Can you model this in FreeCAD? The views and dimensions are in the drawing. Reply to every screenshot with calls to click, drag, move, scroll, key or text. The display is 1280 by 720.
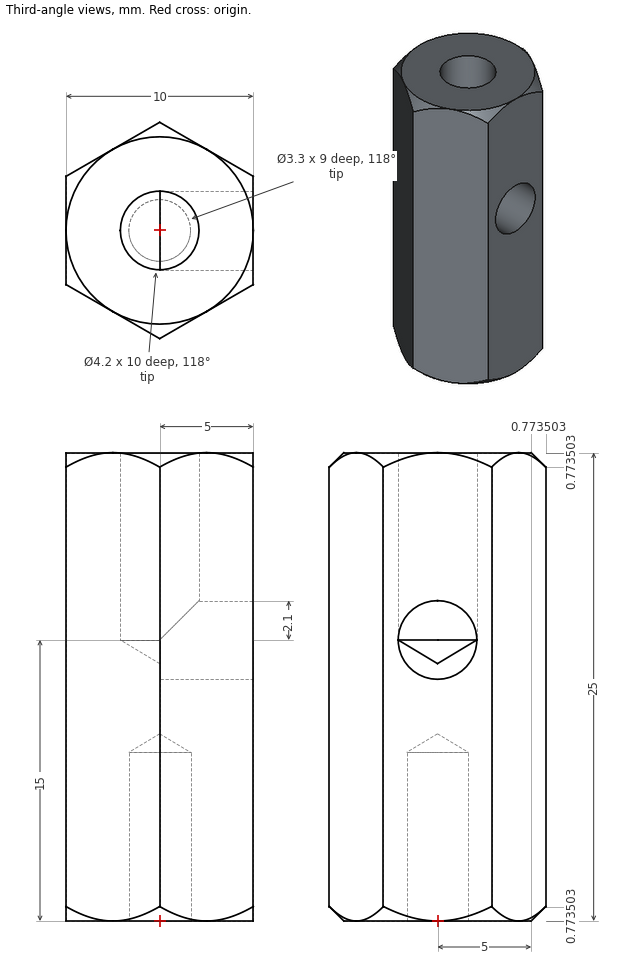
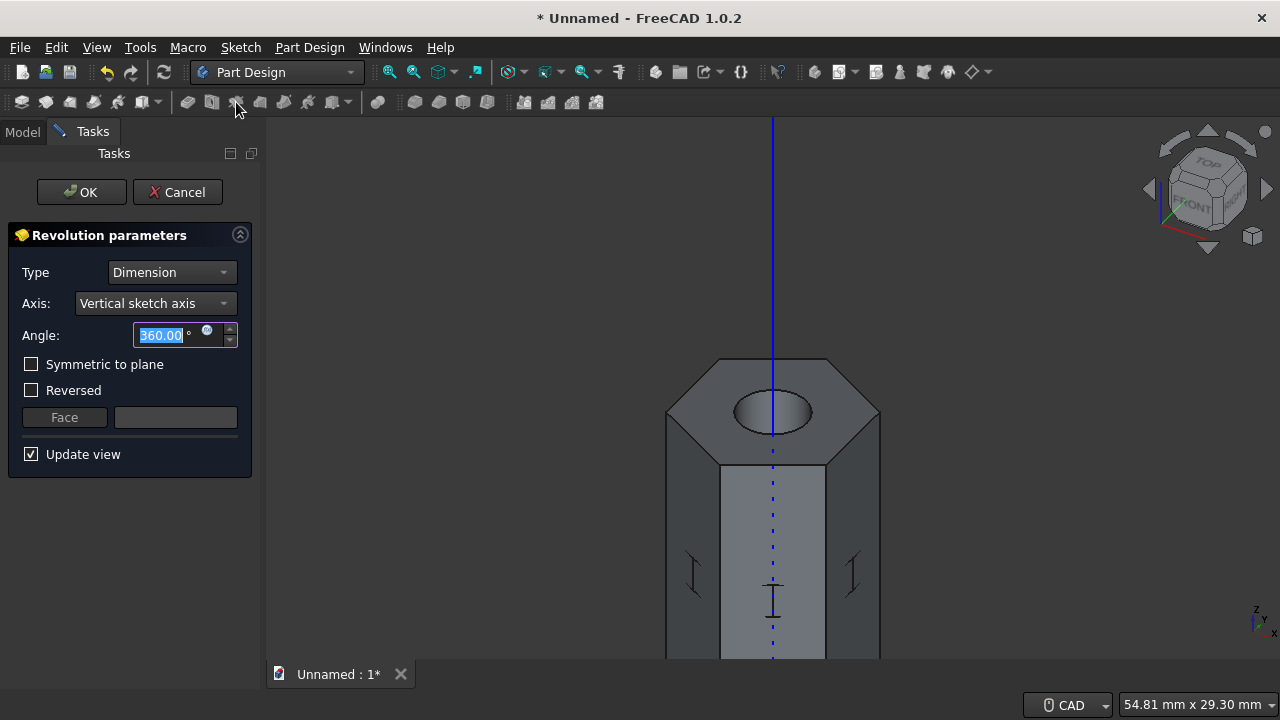
click(156, 304)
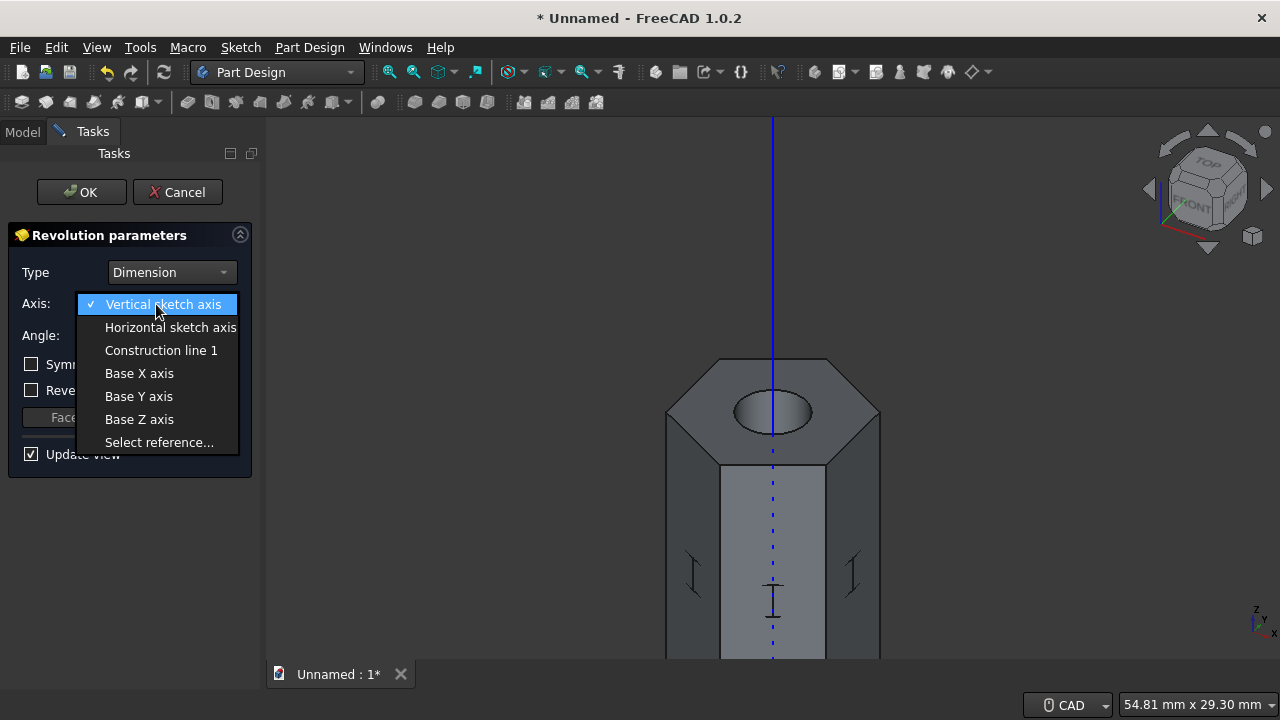
click(156, 350)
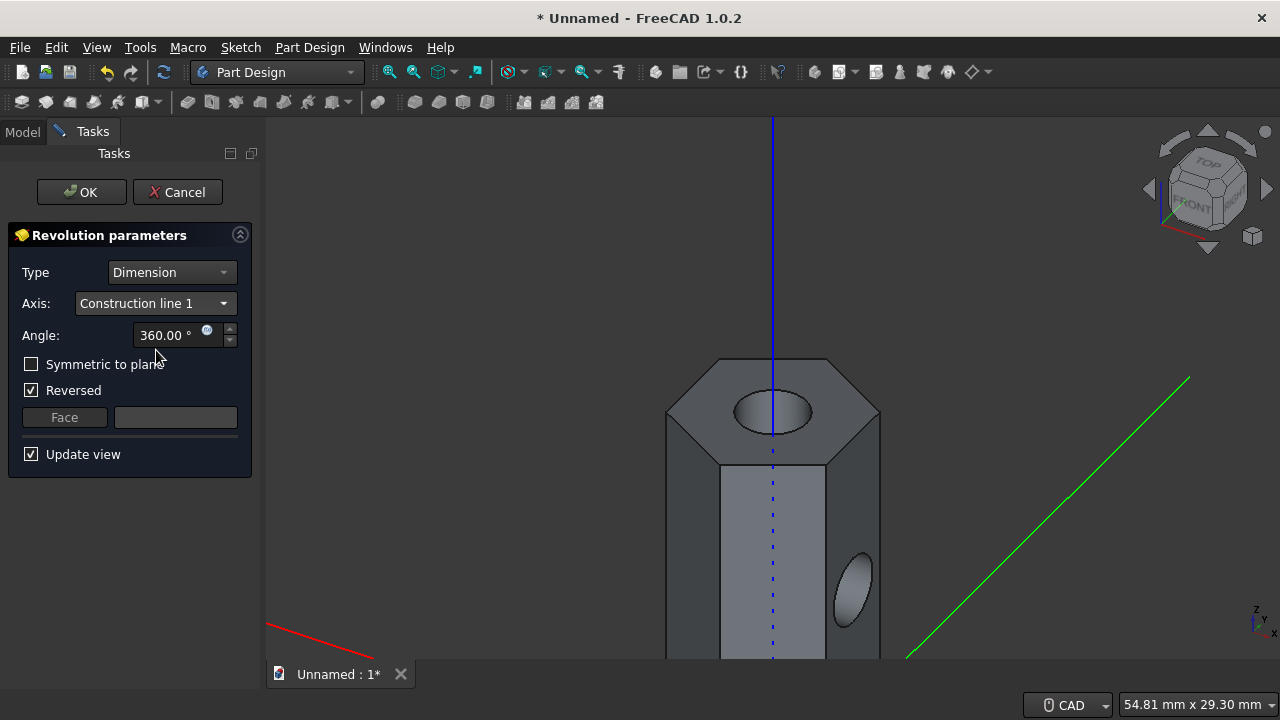
click(82, 192)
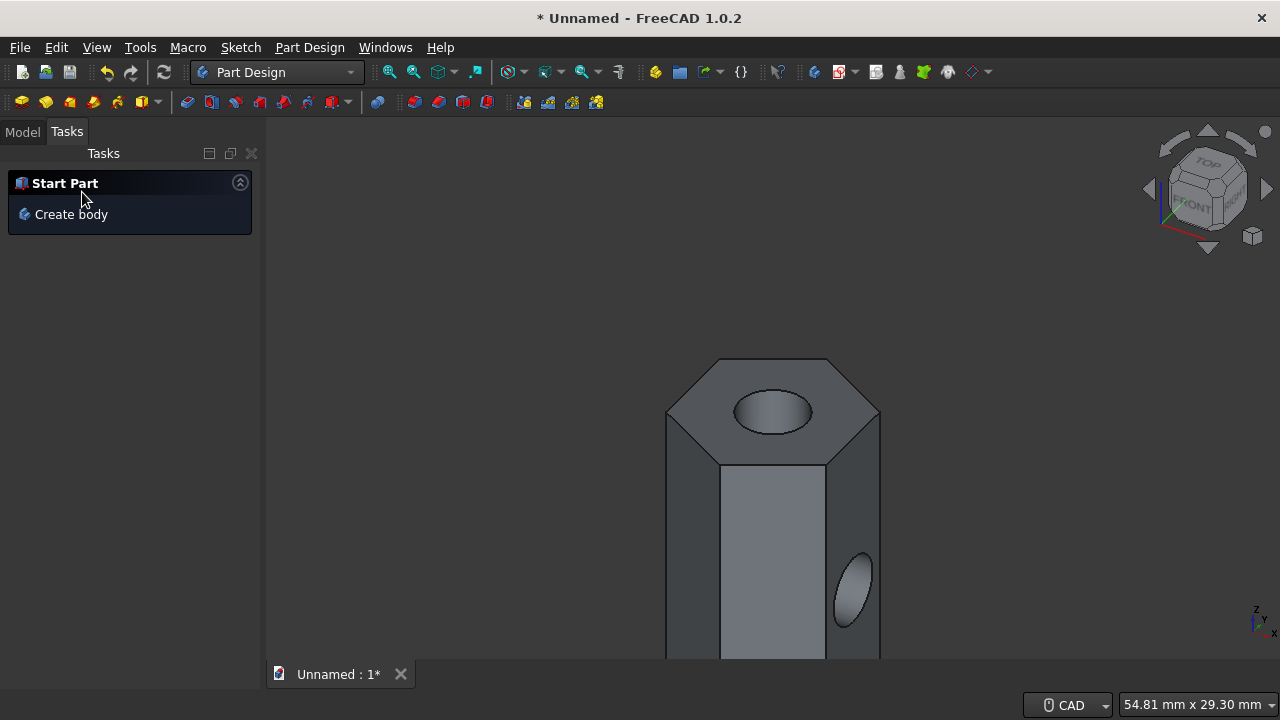
click(390, 72)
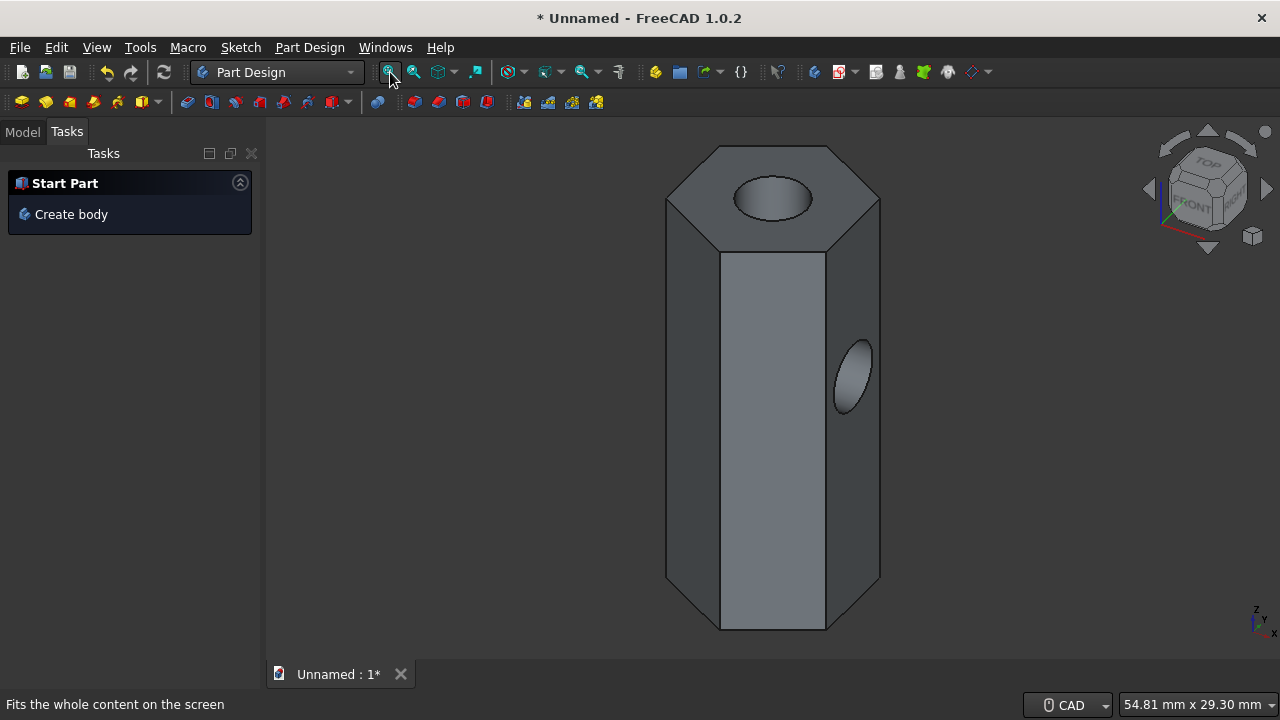
key(0)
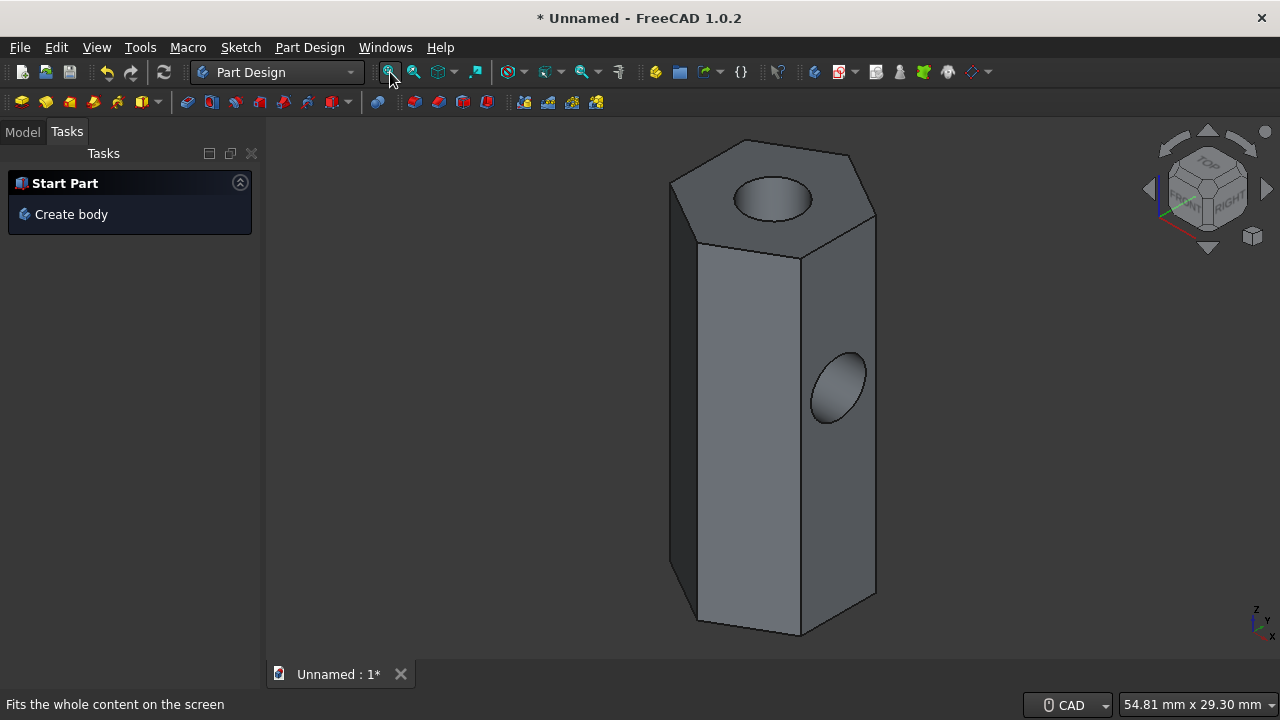
key(3)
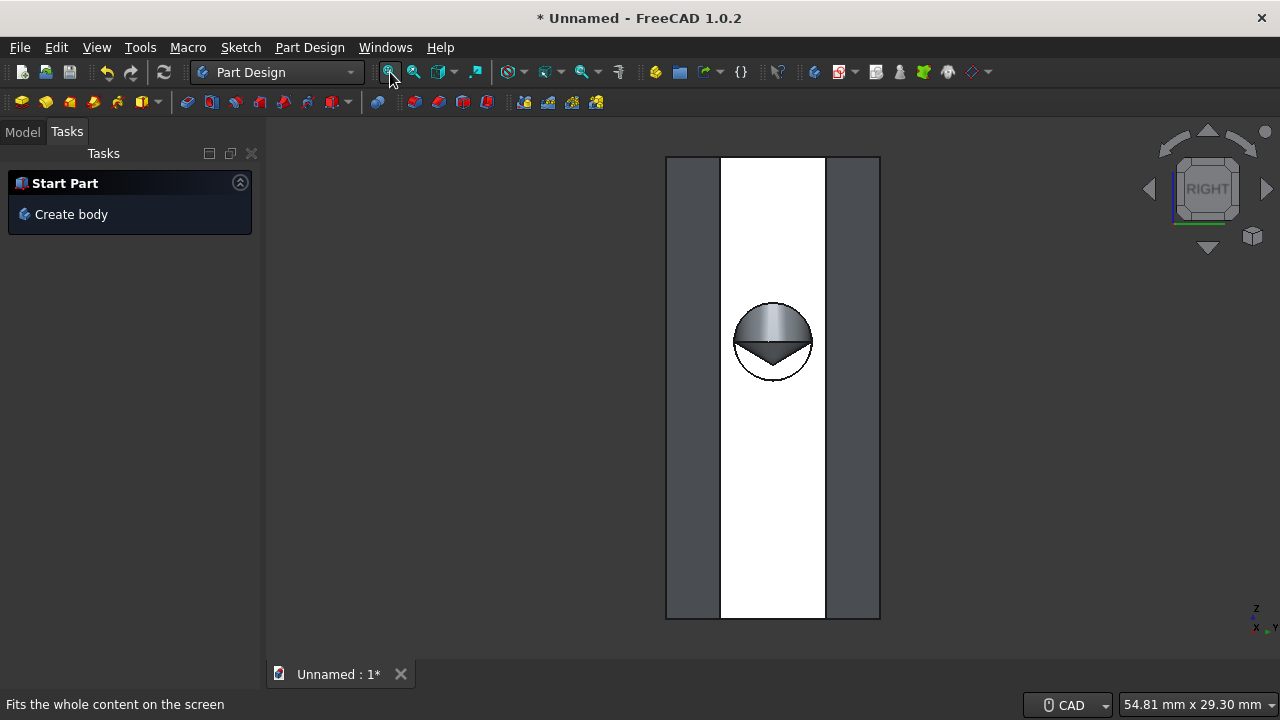
click(795, 360)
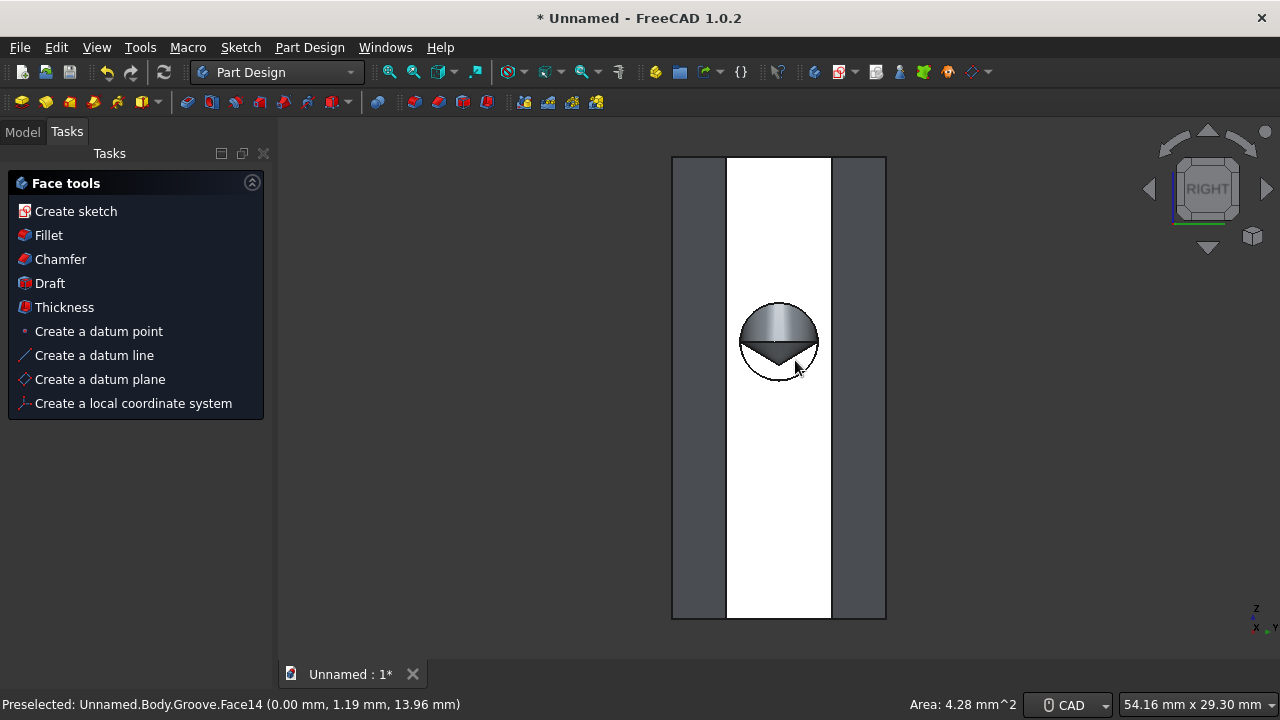
click(840, 72)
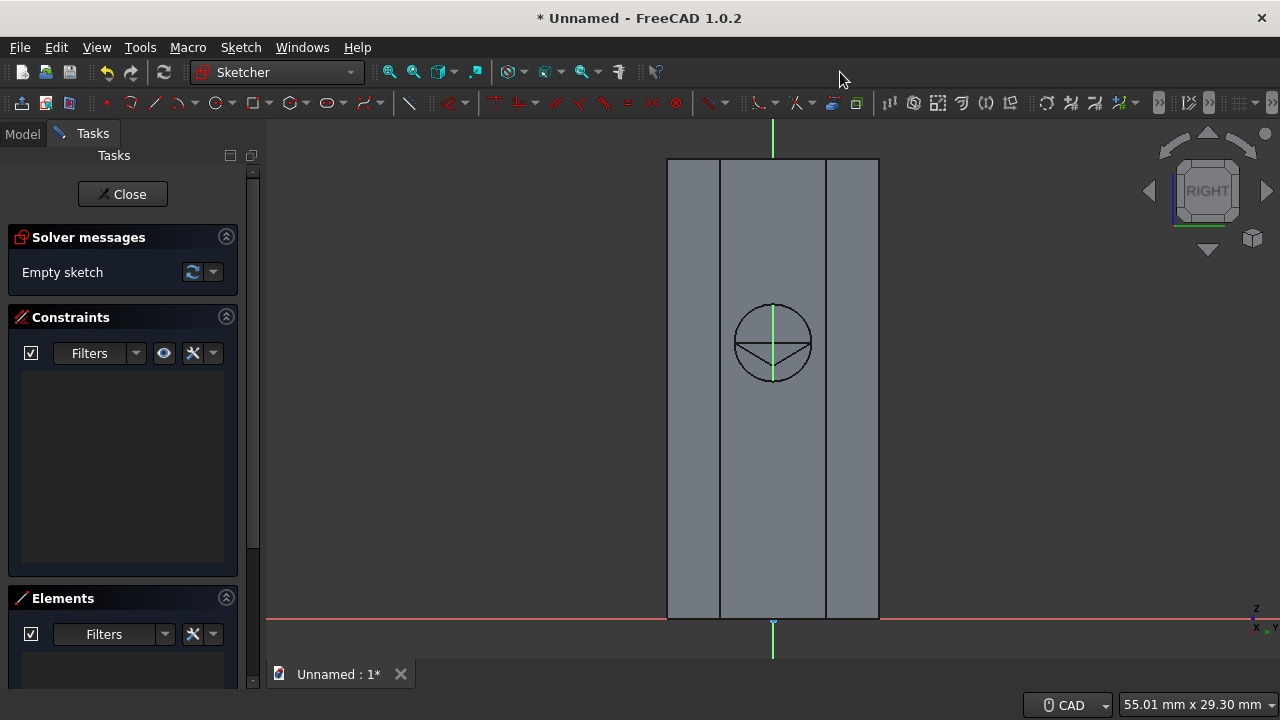
click(70, 104)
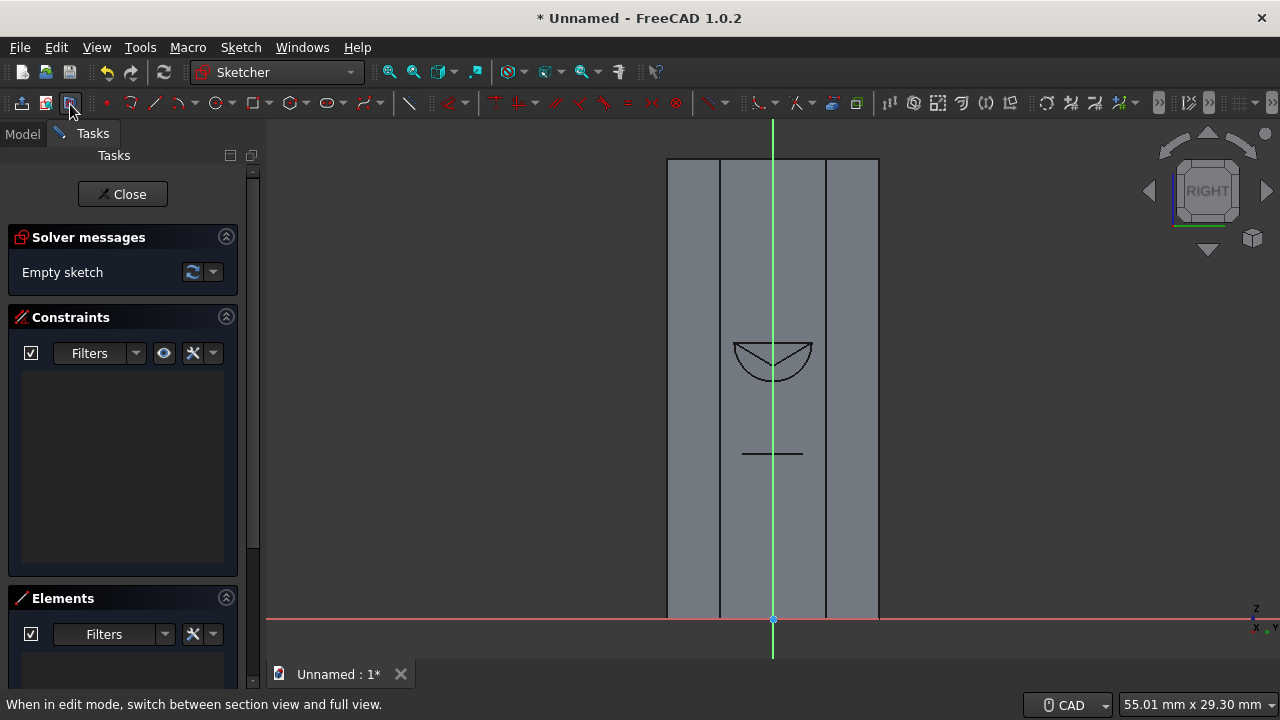
scroll(294, 389, down, 1)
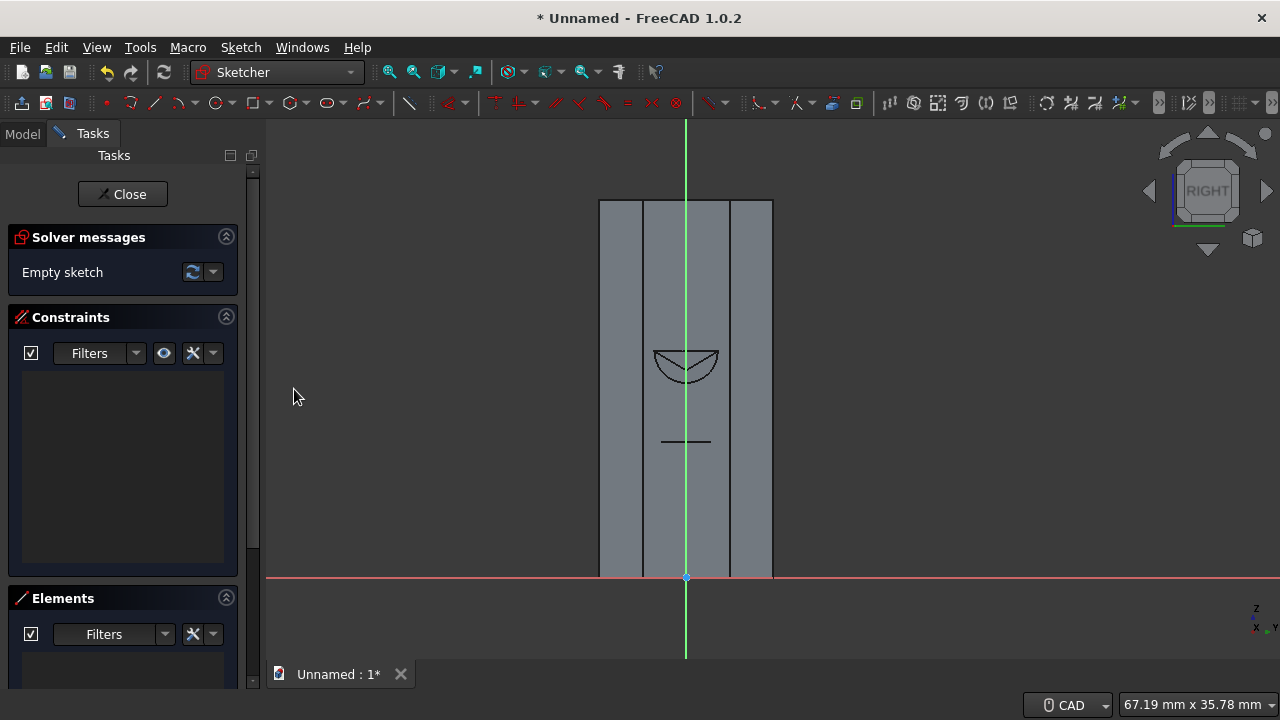
click(132, 104)